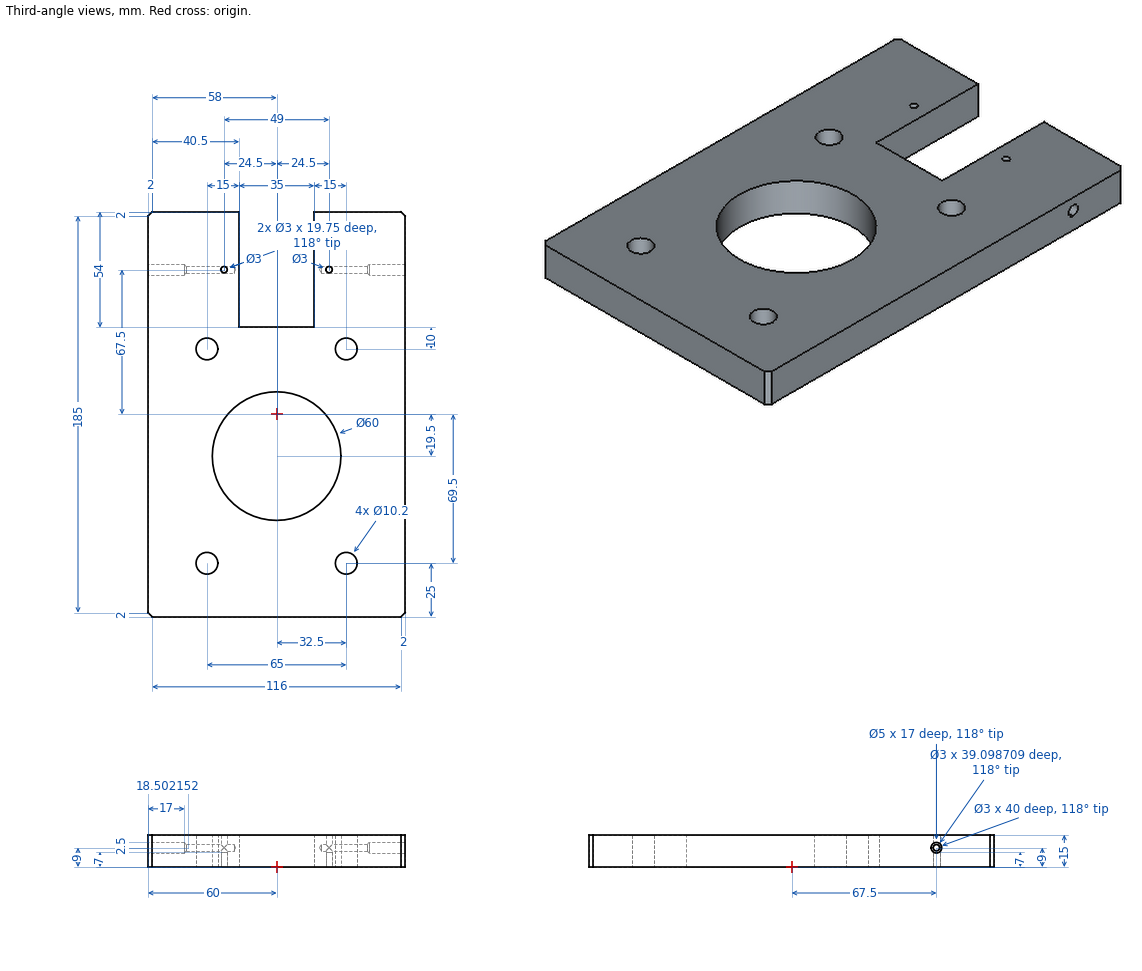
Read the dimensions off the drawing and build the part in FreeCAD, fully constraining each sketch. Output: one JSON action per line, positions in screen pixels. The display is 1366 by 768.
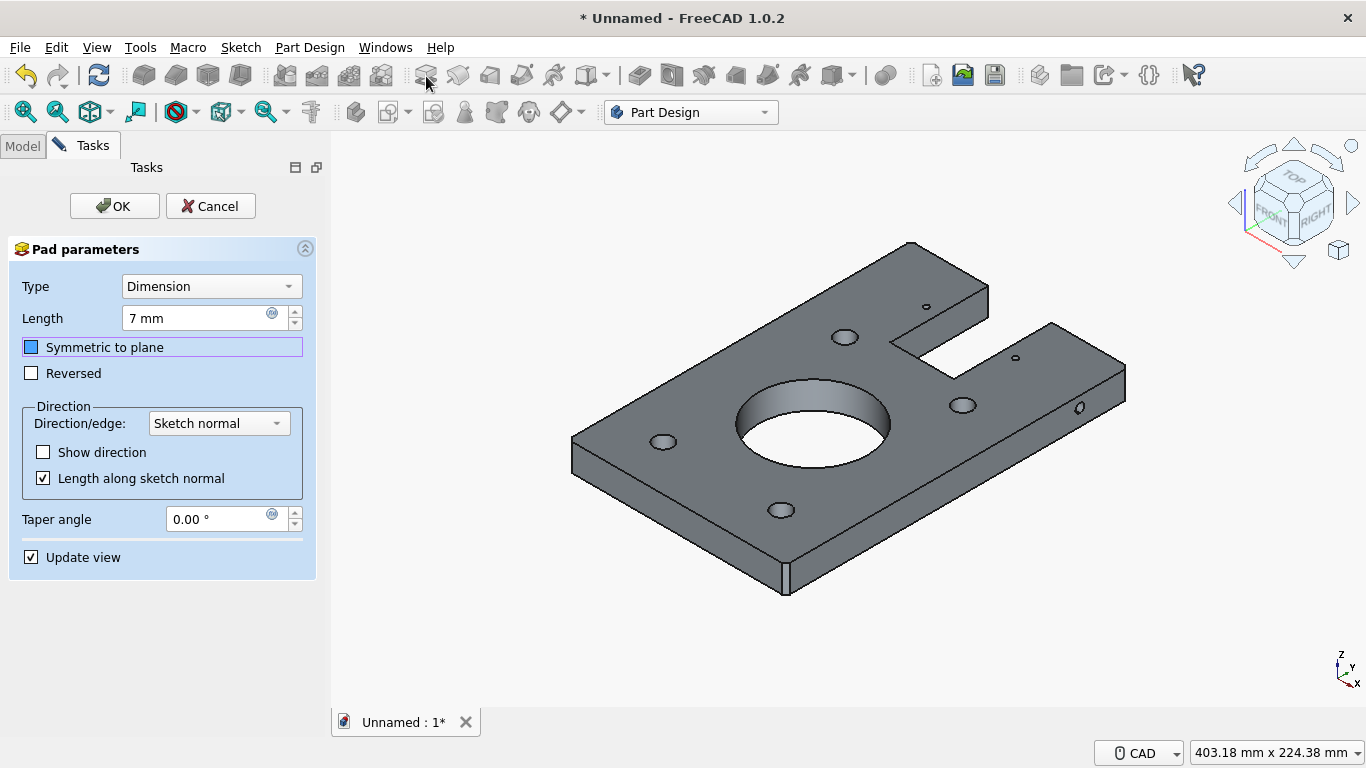
{"action": "left_click", "coordinate": [115, 206]}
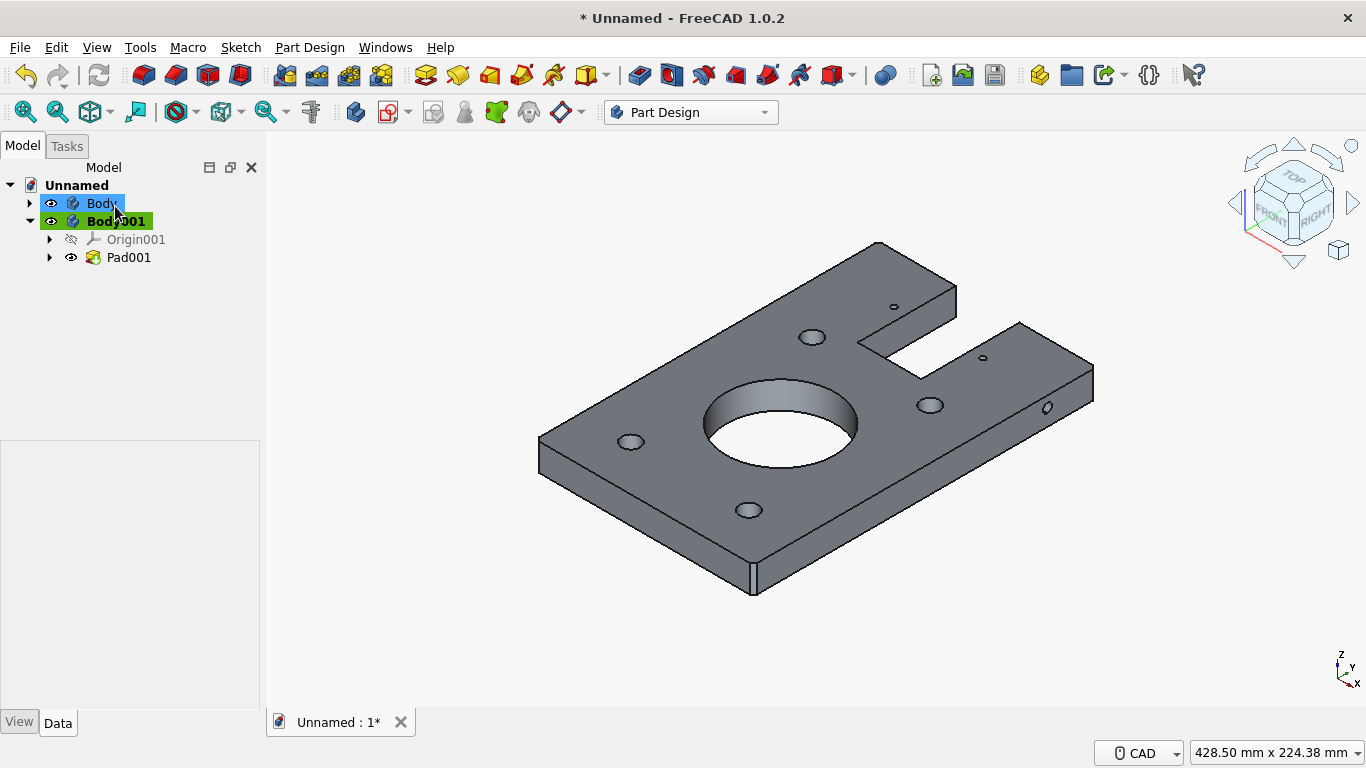
{"action": "left_click", "coordinate": [26, 112]}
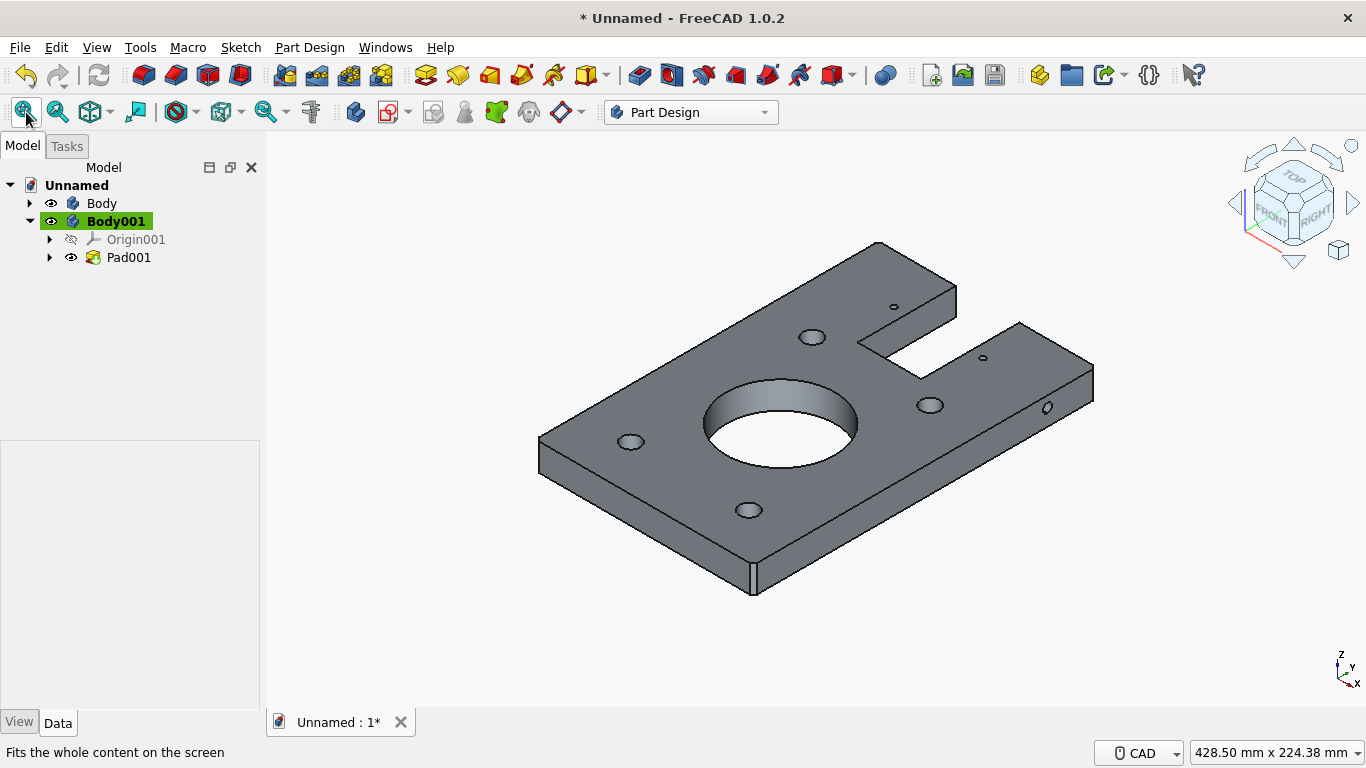
{"action": "left_click", "coordinate": [356, 112]}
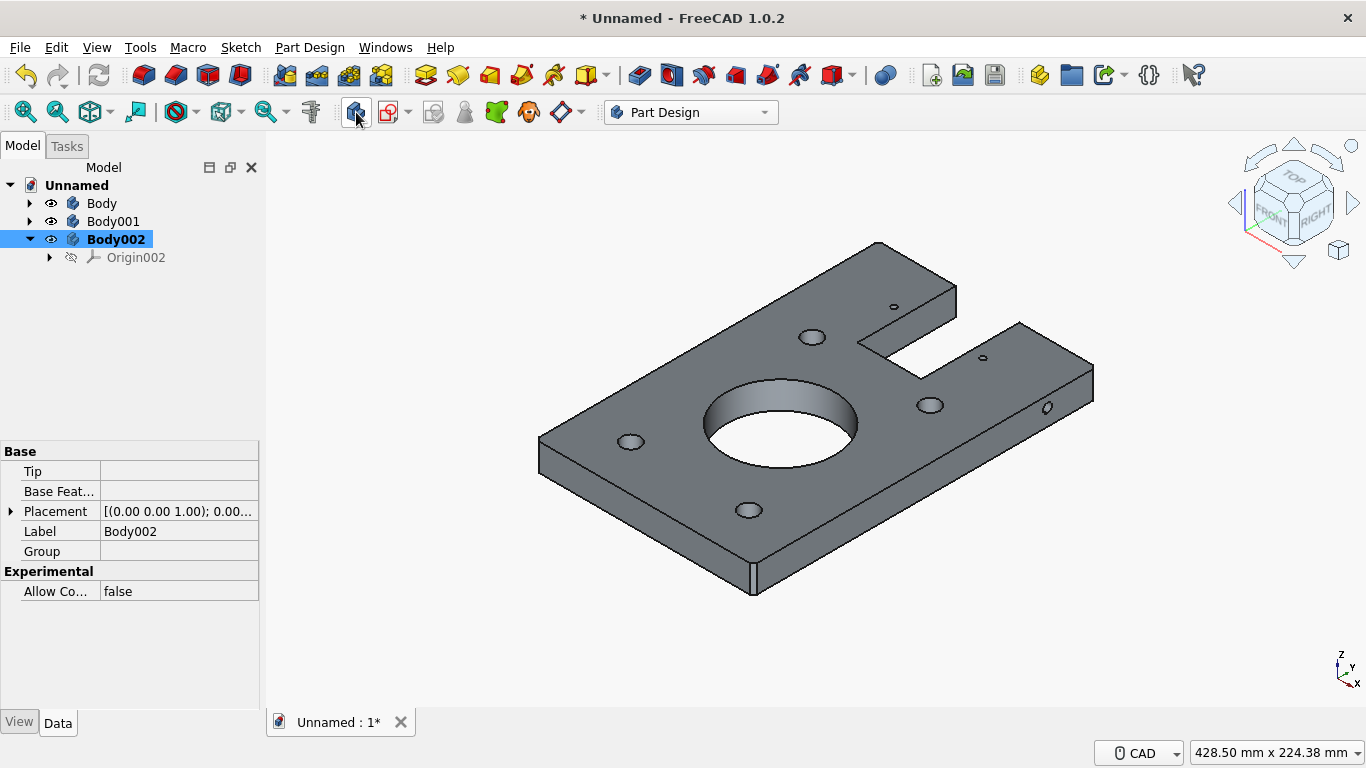
{"action": "left_click", "coordinate": [306, 667]}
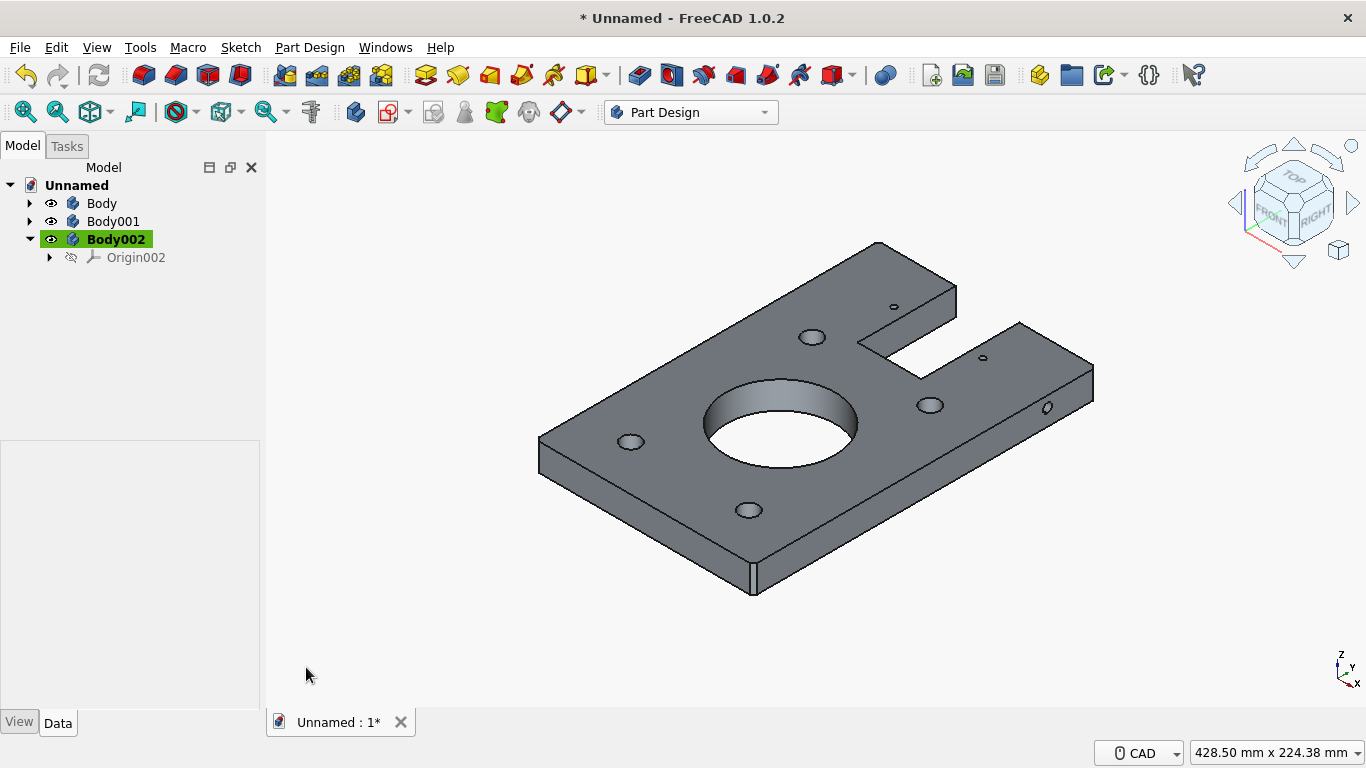
{"action": "left_click", "coordinate": [388, 112]}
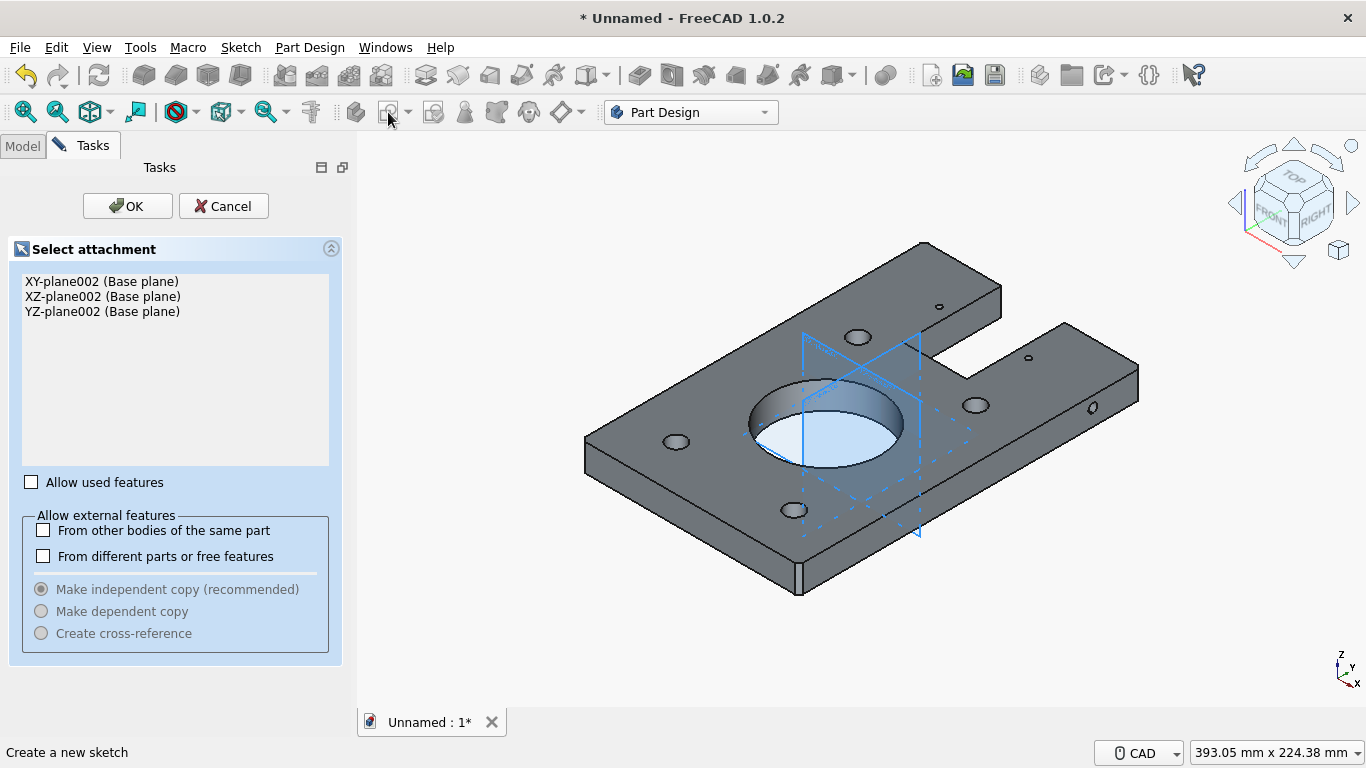
{"action": "left_click", "coordinate": [82, 282]}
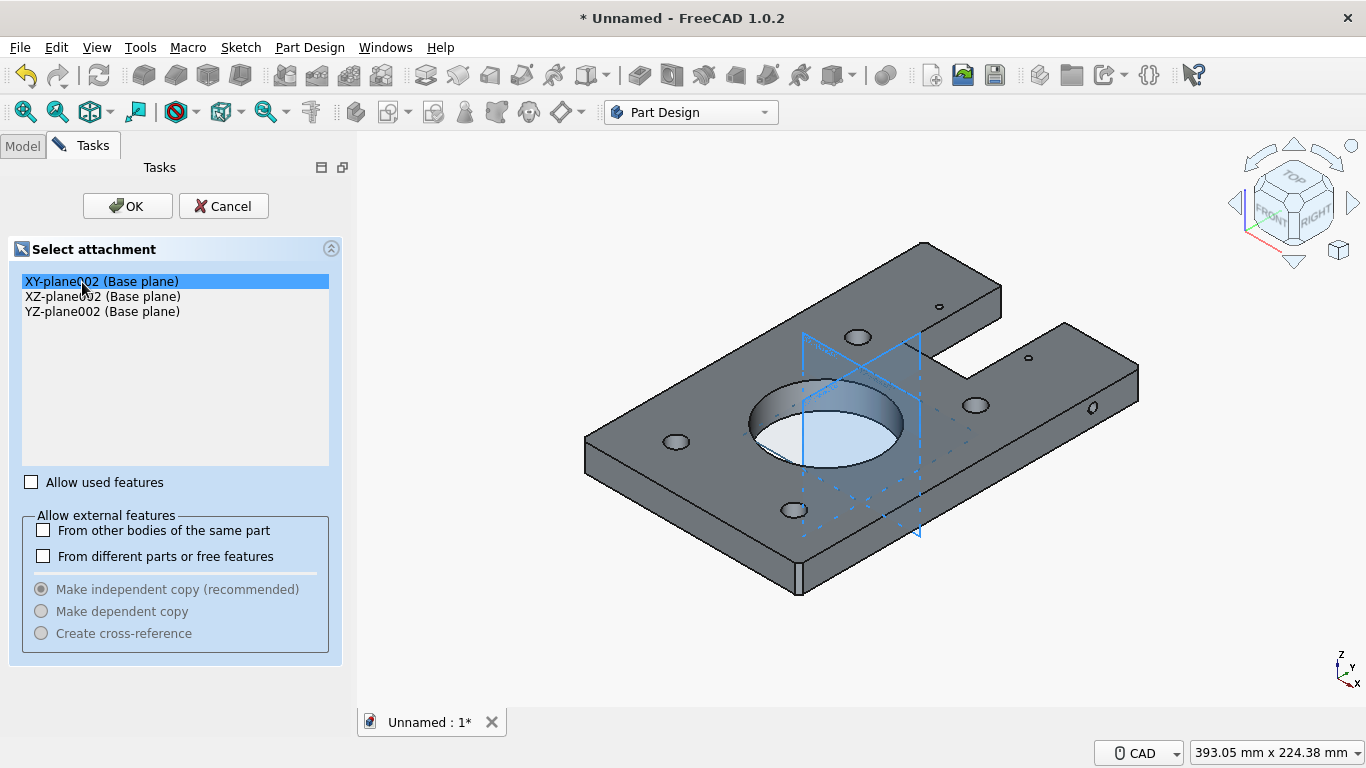
{"action": "left_click", "coordinate": [128, 206]}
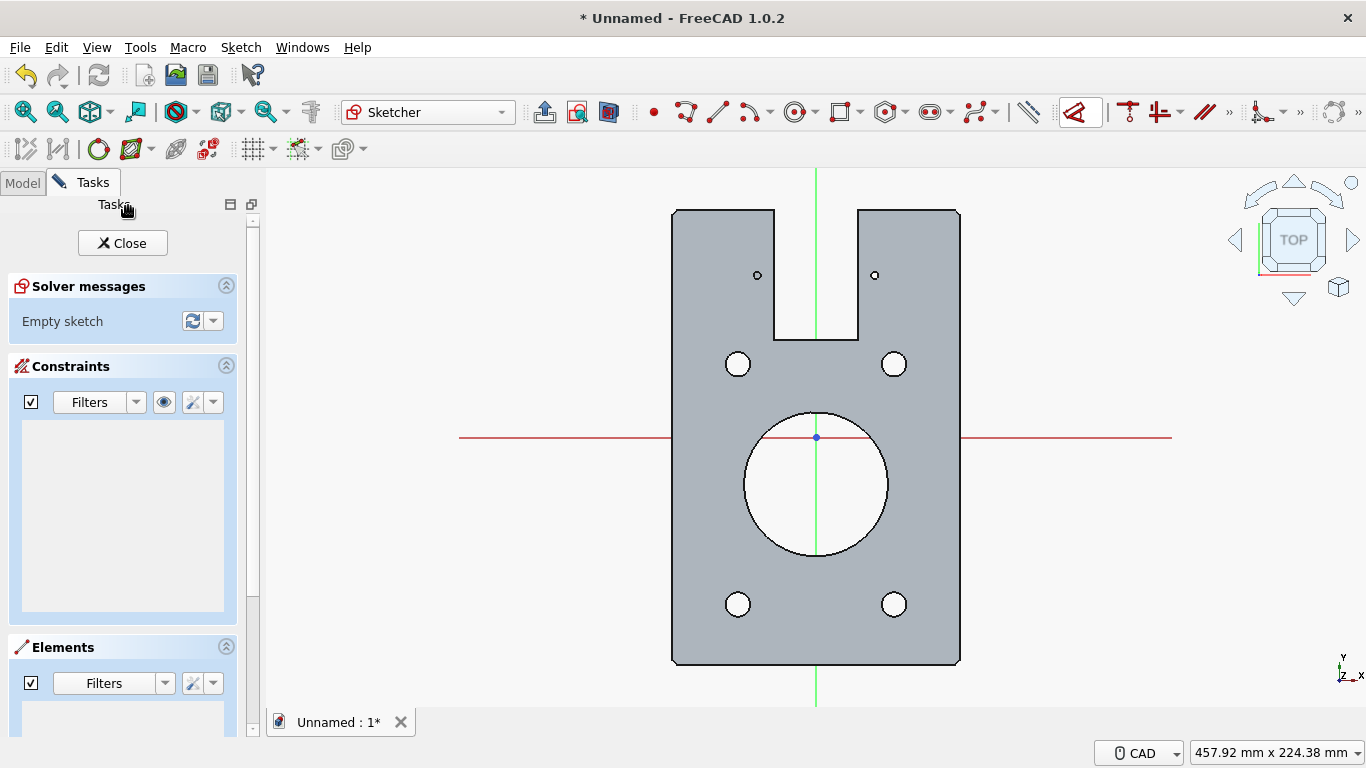
{"action": "scroll", "coordinate": [882, 267], "scroll_direction": "up", "scroll_amount": 15}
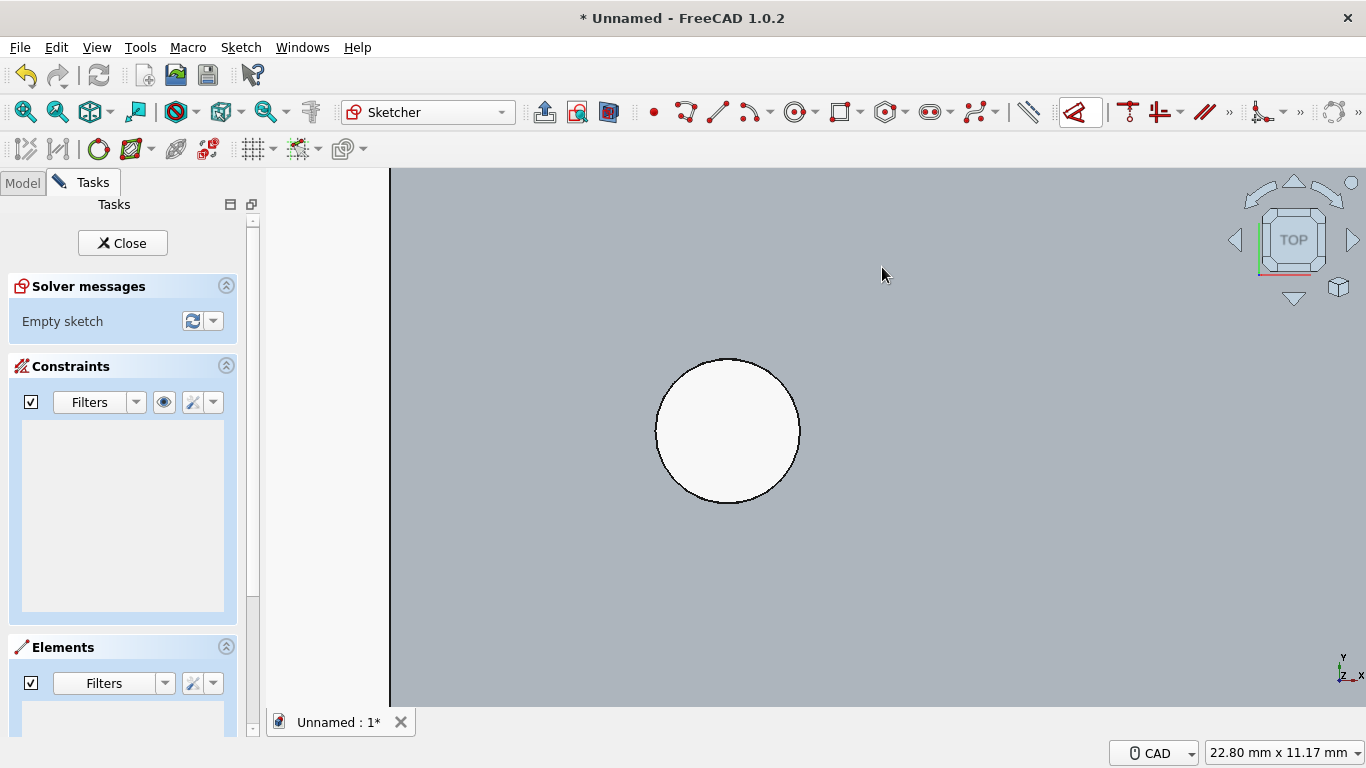
{"action": "scroll", "coordinate": [712, 426], "scroll_direction": "up", "scroll_amount": 4}